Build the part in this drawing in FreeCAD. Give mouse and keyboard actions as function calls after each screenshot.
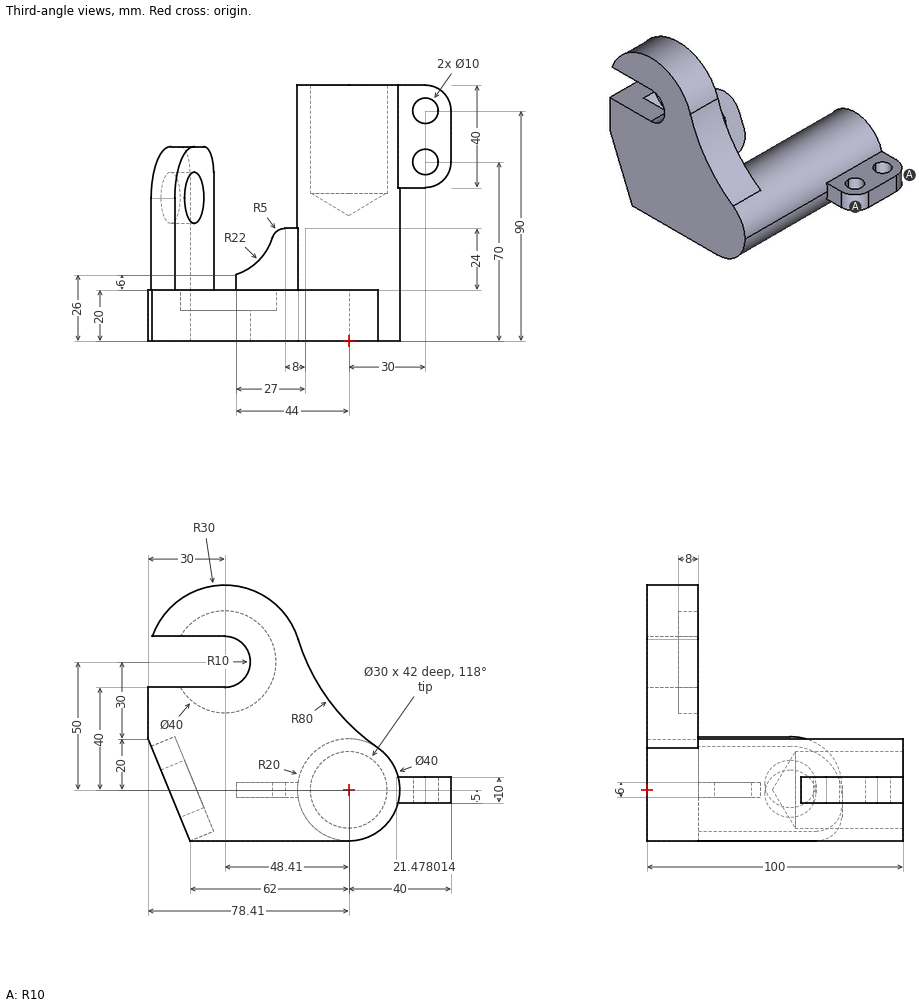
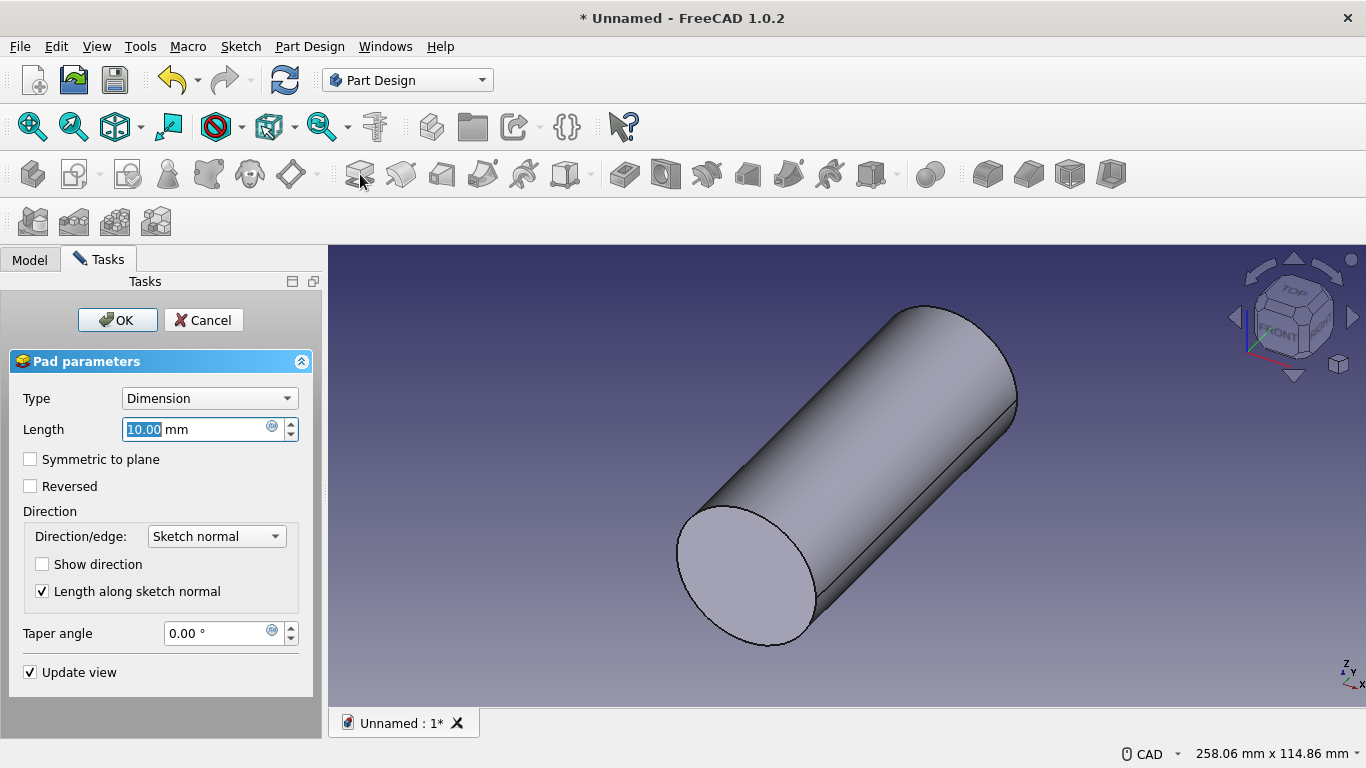
text(20)
key(Tab)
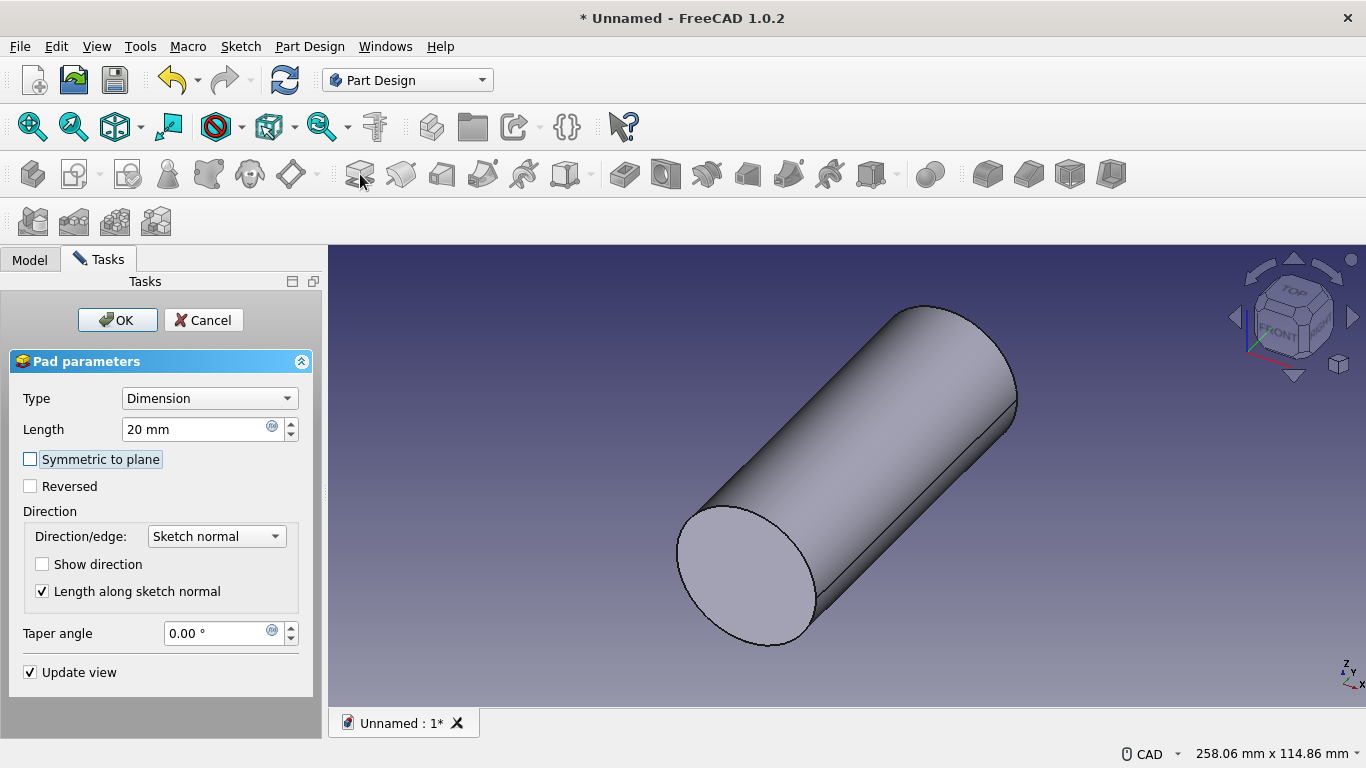
click(31, 486)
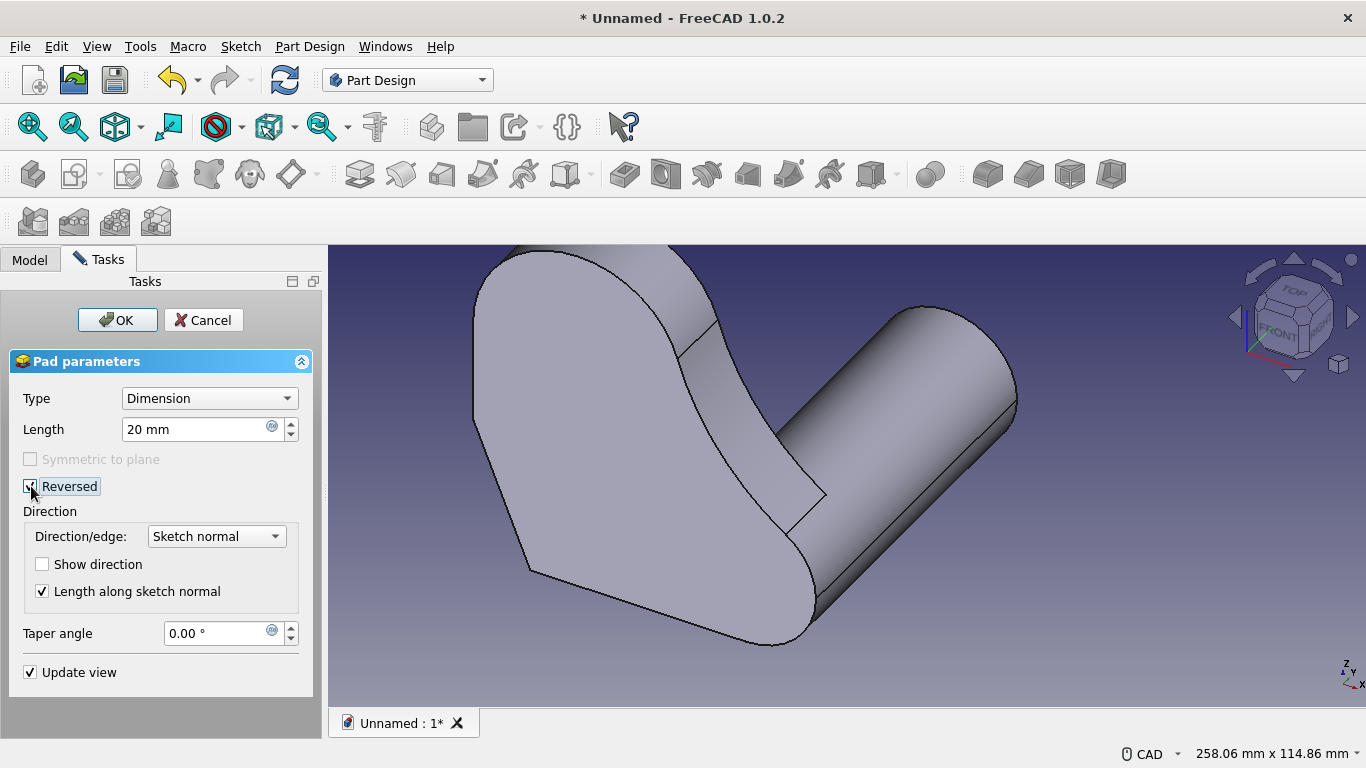
click(118, 320)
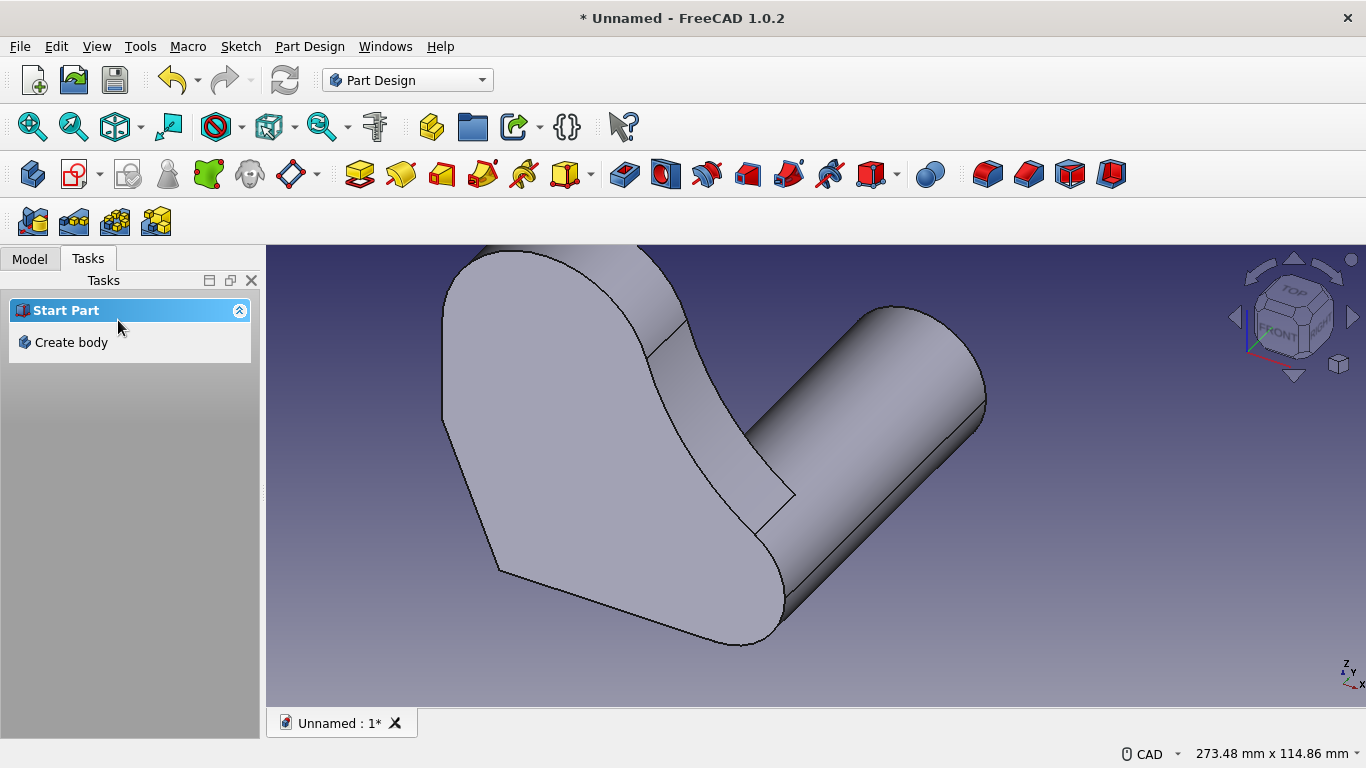
key(v)
key(f)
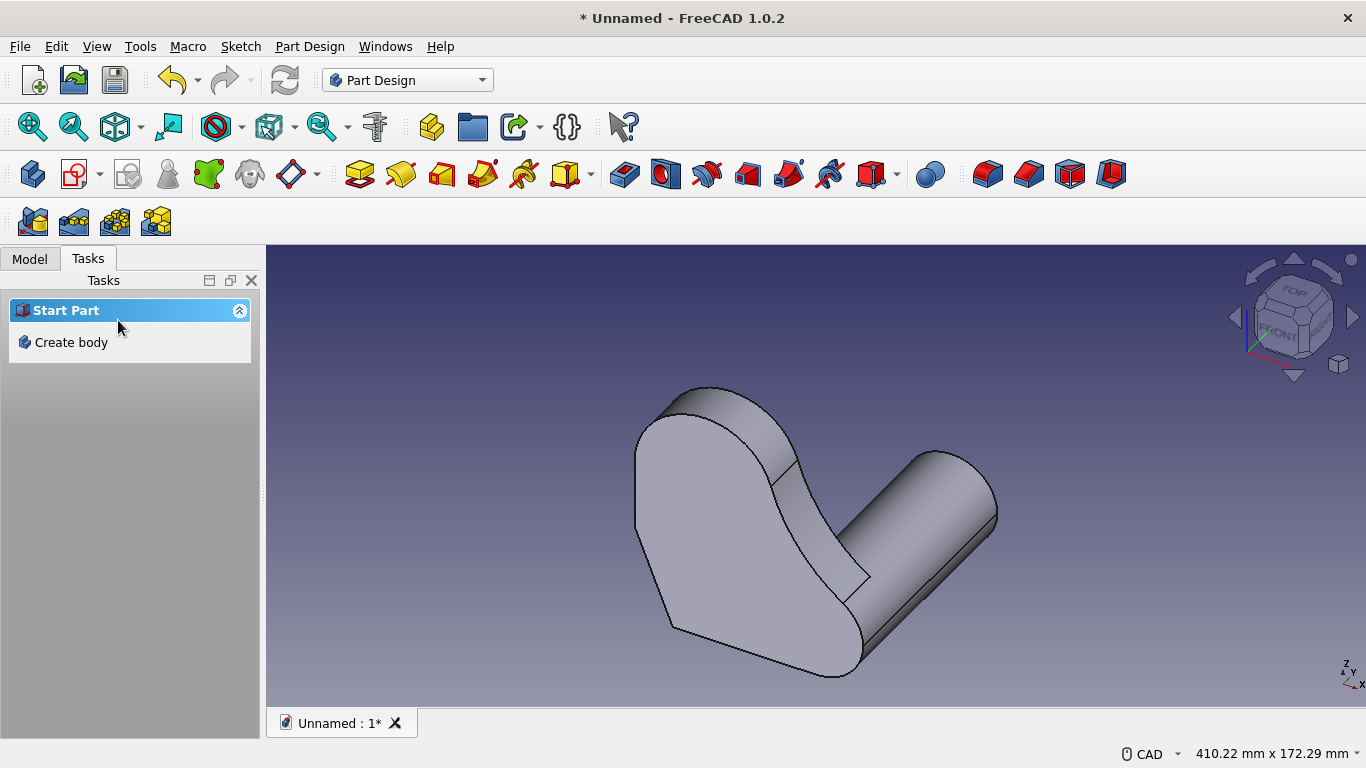
key(4)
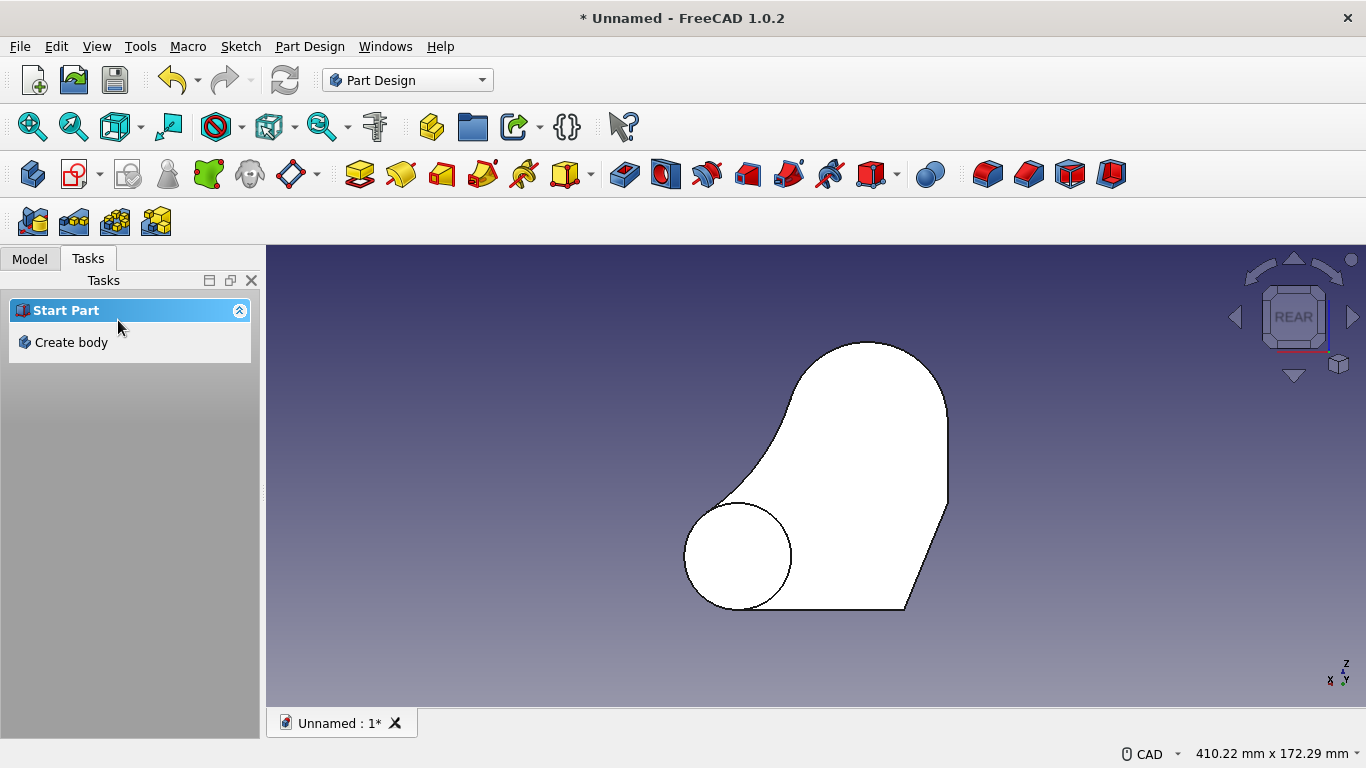
click(738, 555)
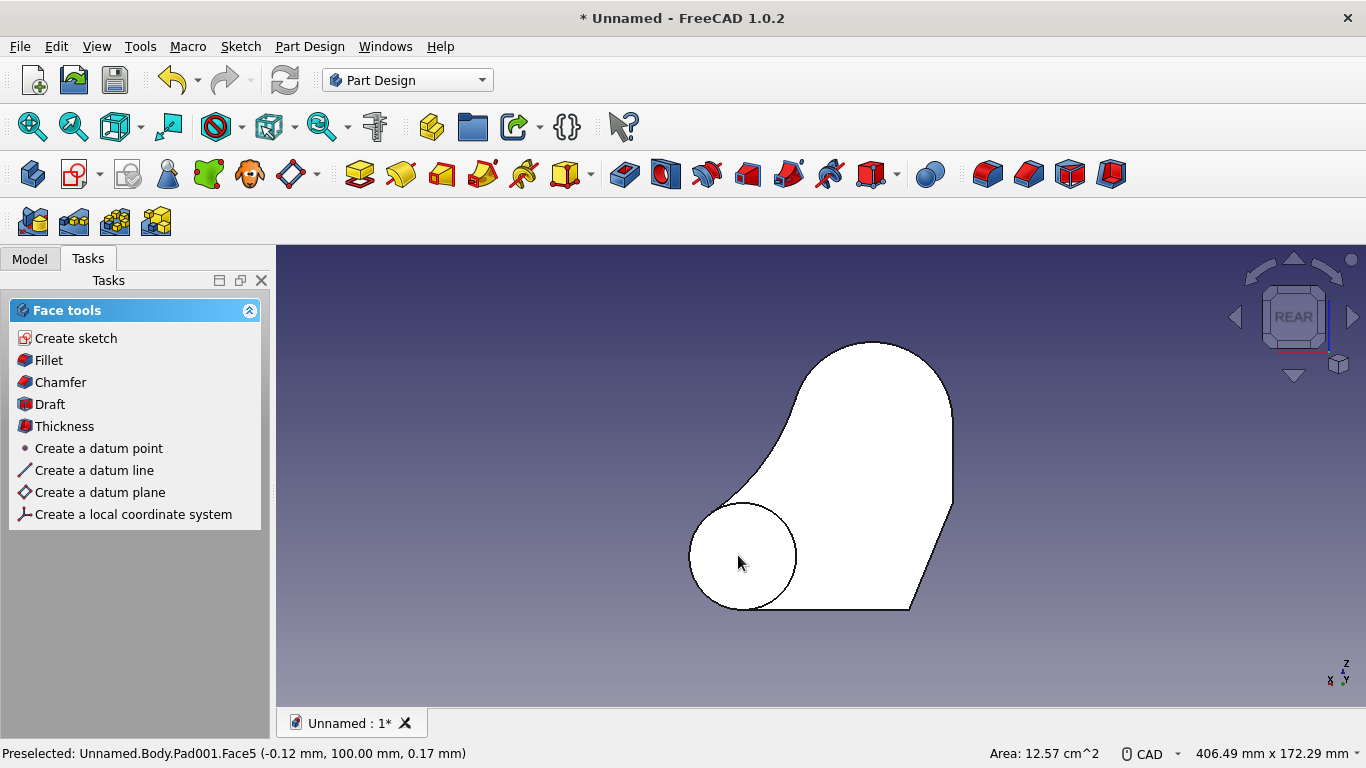
click(74, 174)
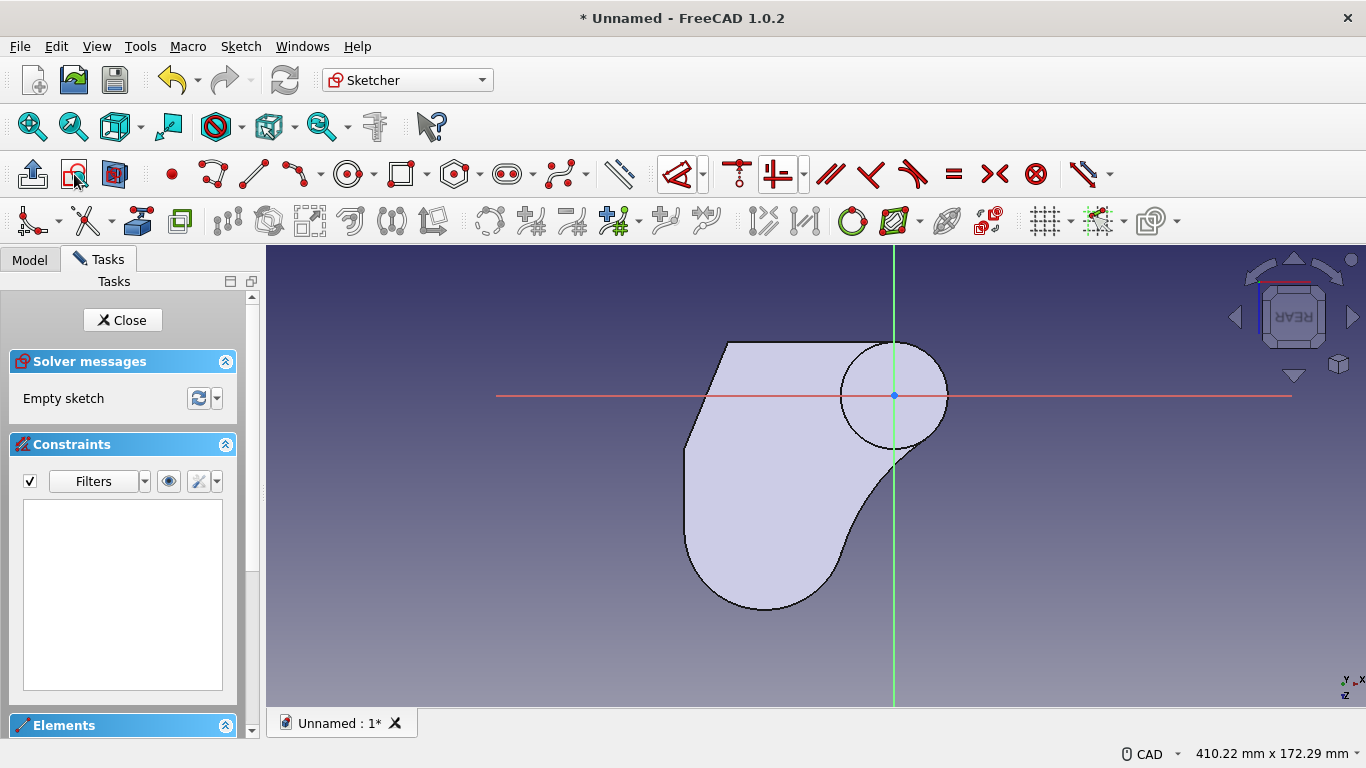
scroll(958, 361, up, 6)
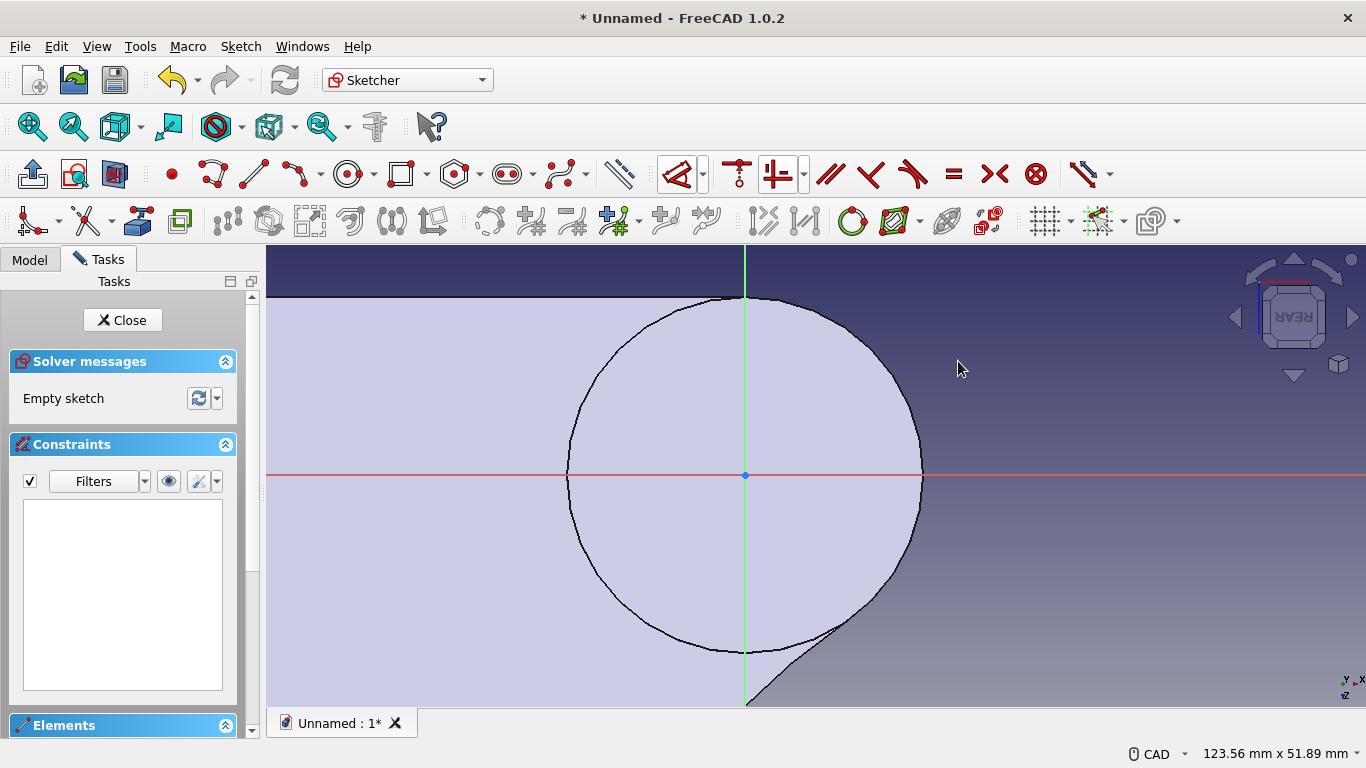
key(g)
key(c)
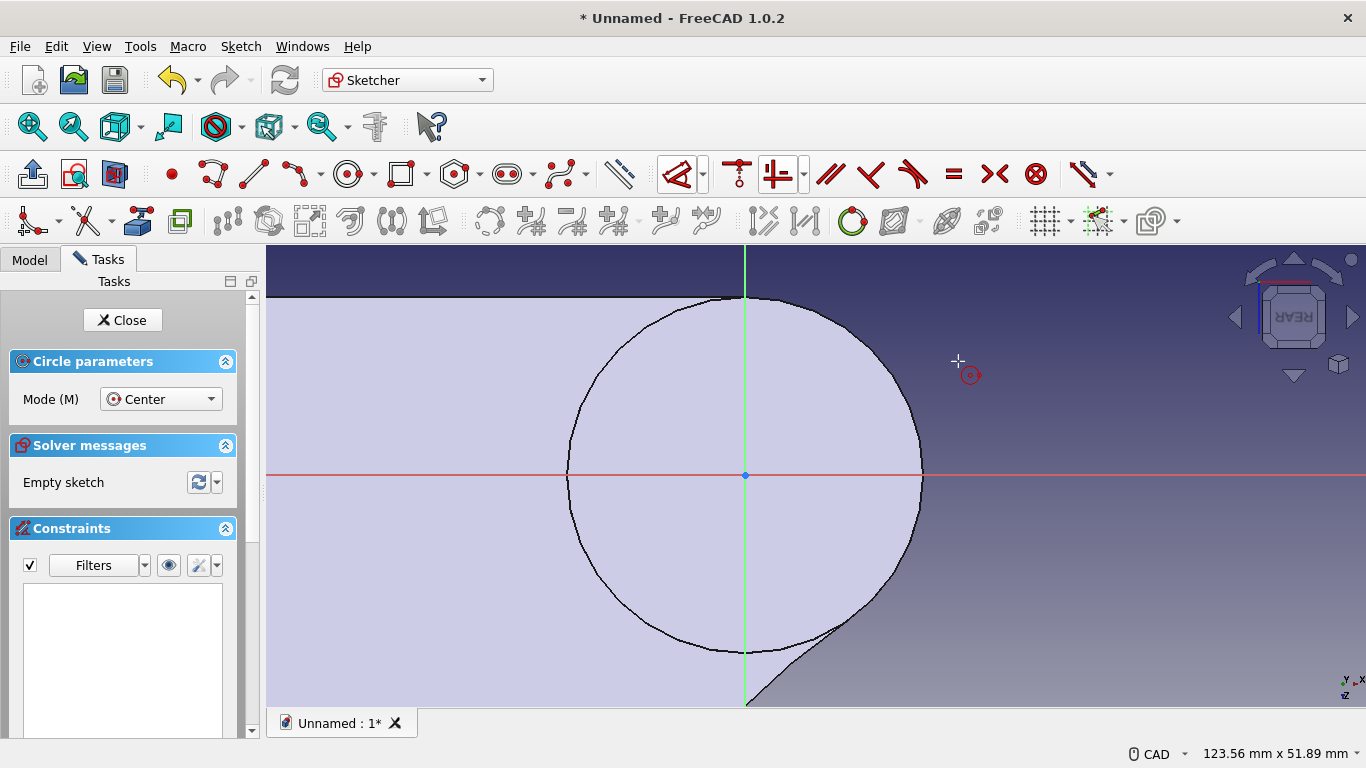
click(745, 475)
click(840, 381)
key(Escape)